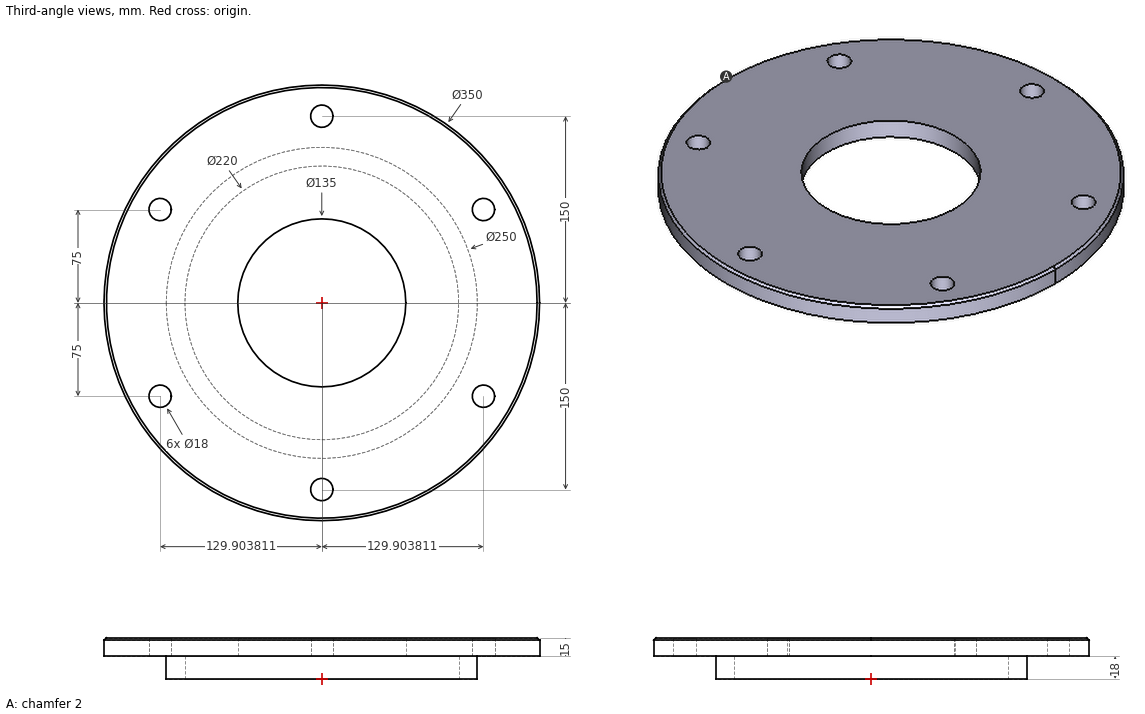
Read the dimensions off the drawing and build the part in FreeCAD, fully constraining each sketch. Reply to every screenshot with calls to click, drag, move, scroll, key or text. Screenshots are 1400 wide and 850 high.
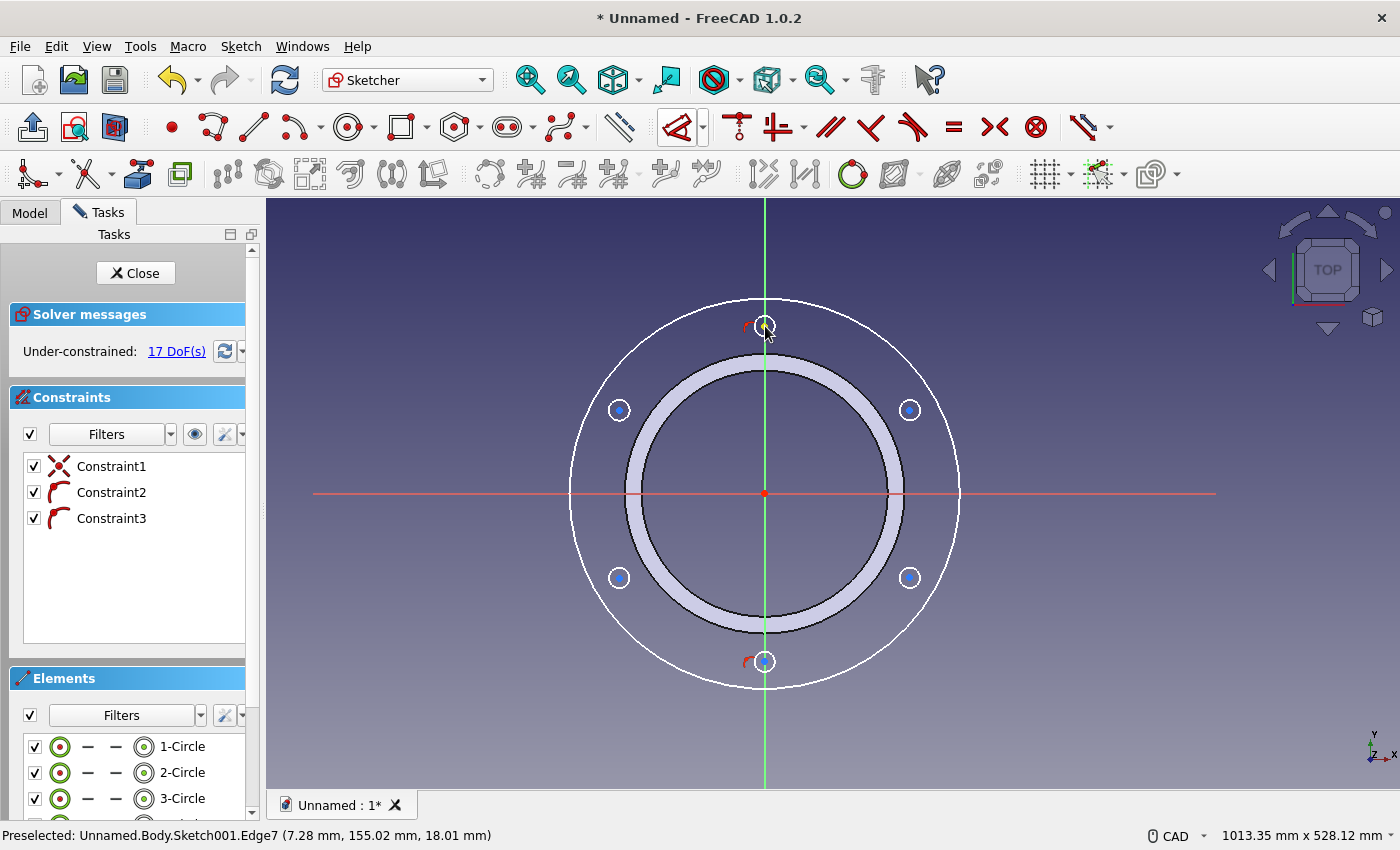
scroll(626, 571, up, 2)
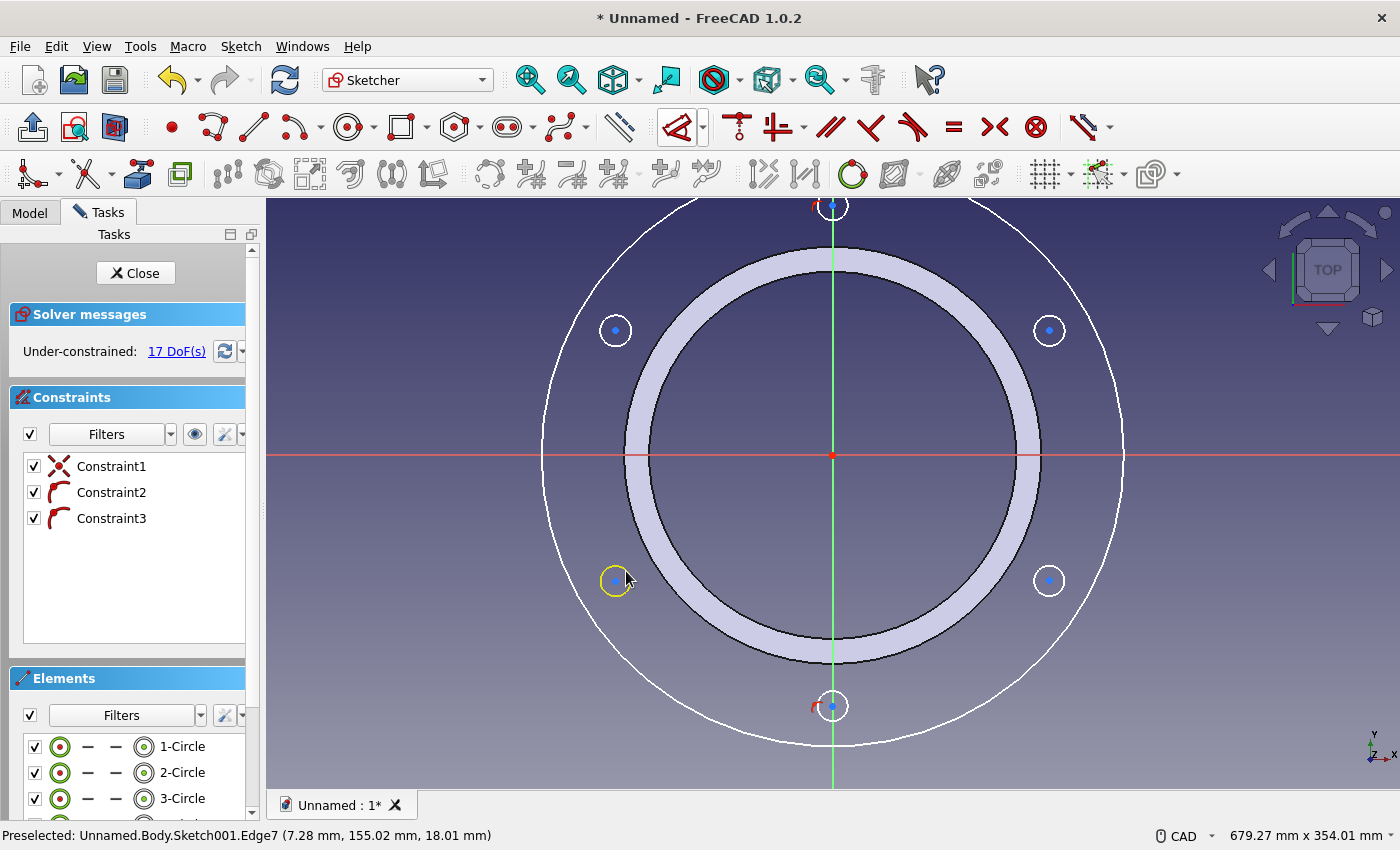
click(626, 570)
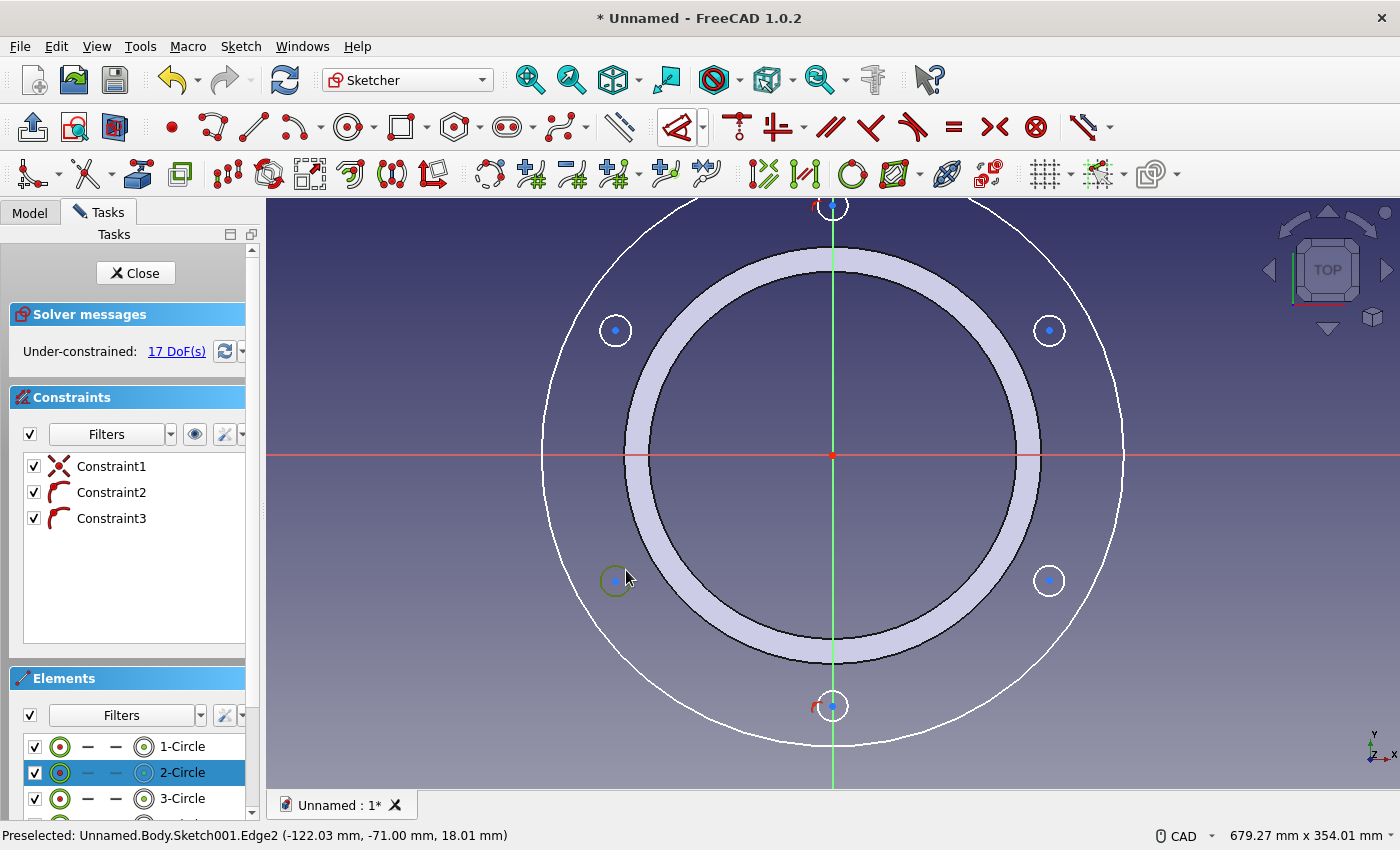
scroll(843, 695, up, 2)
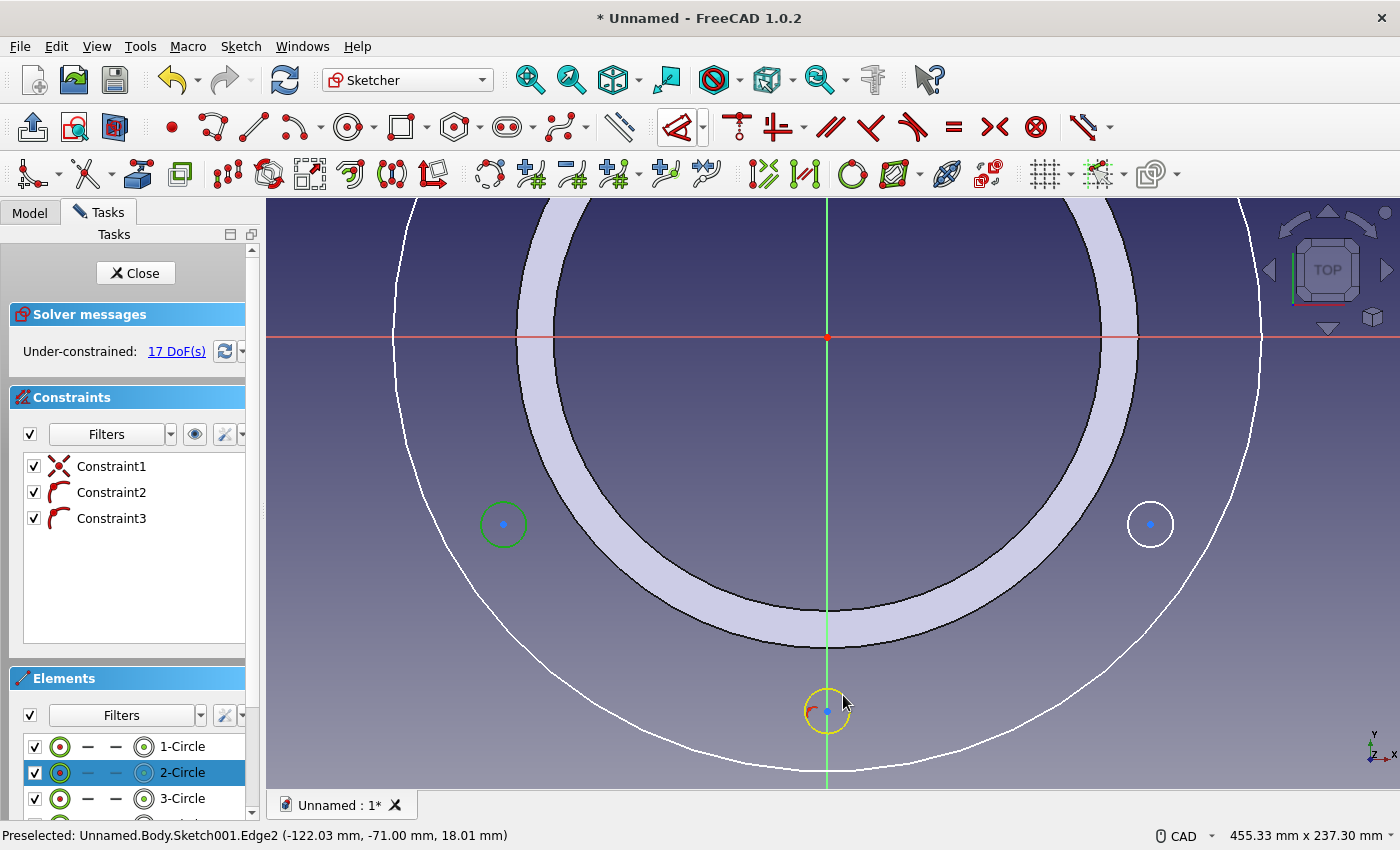
click(843, 695)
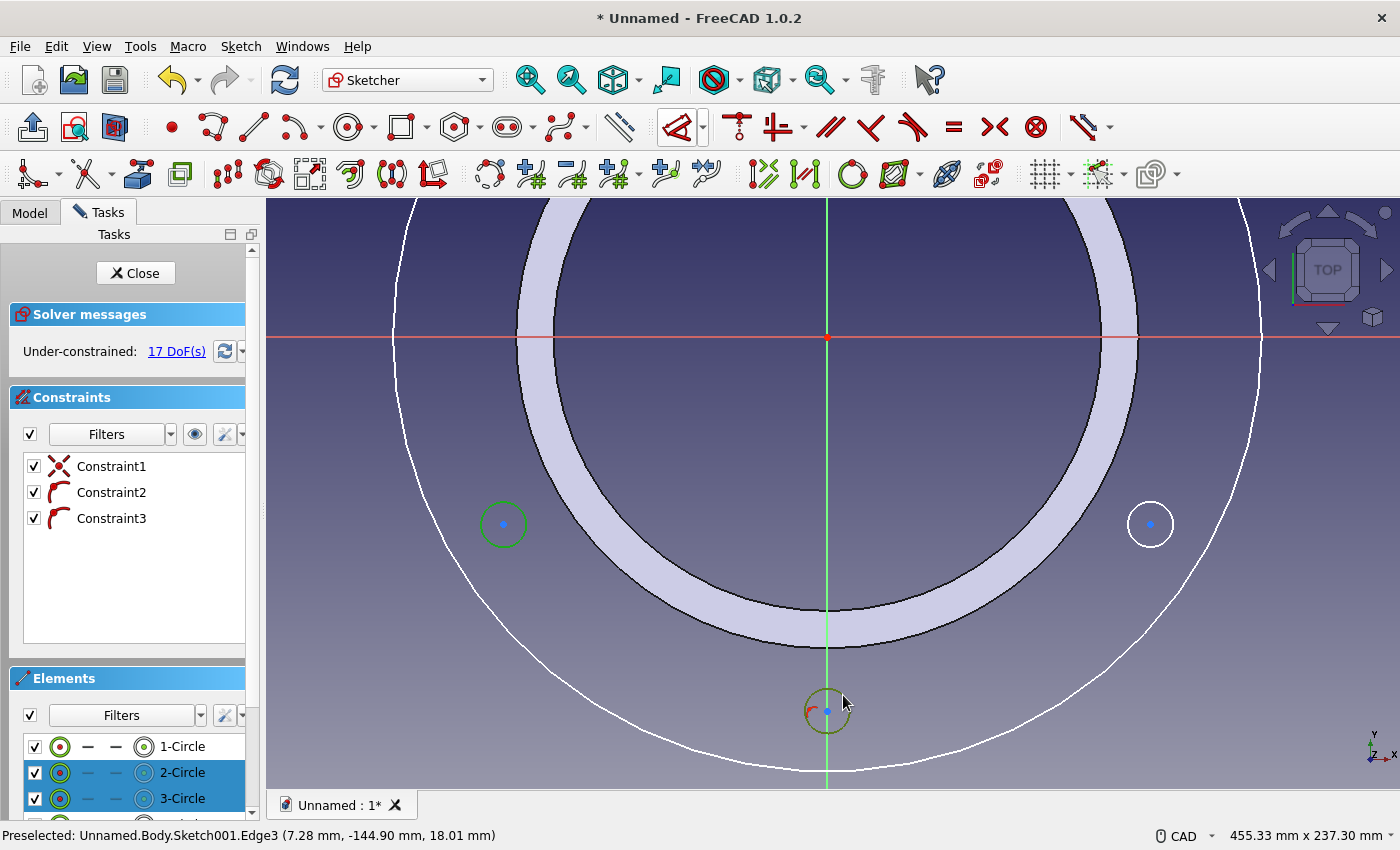
click(1166, 508)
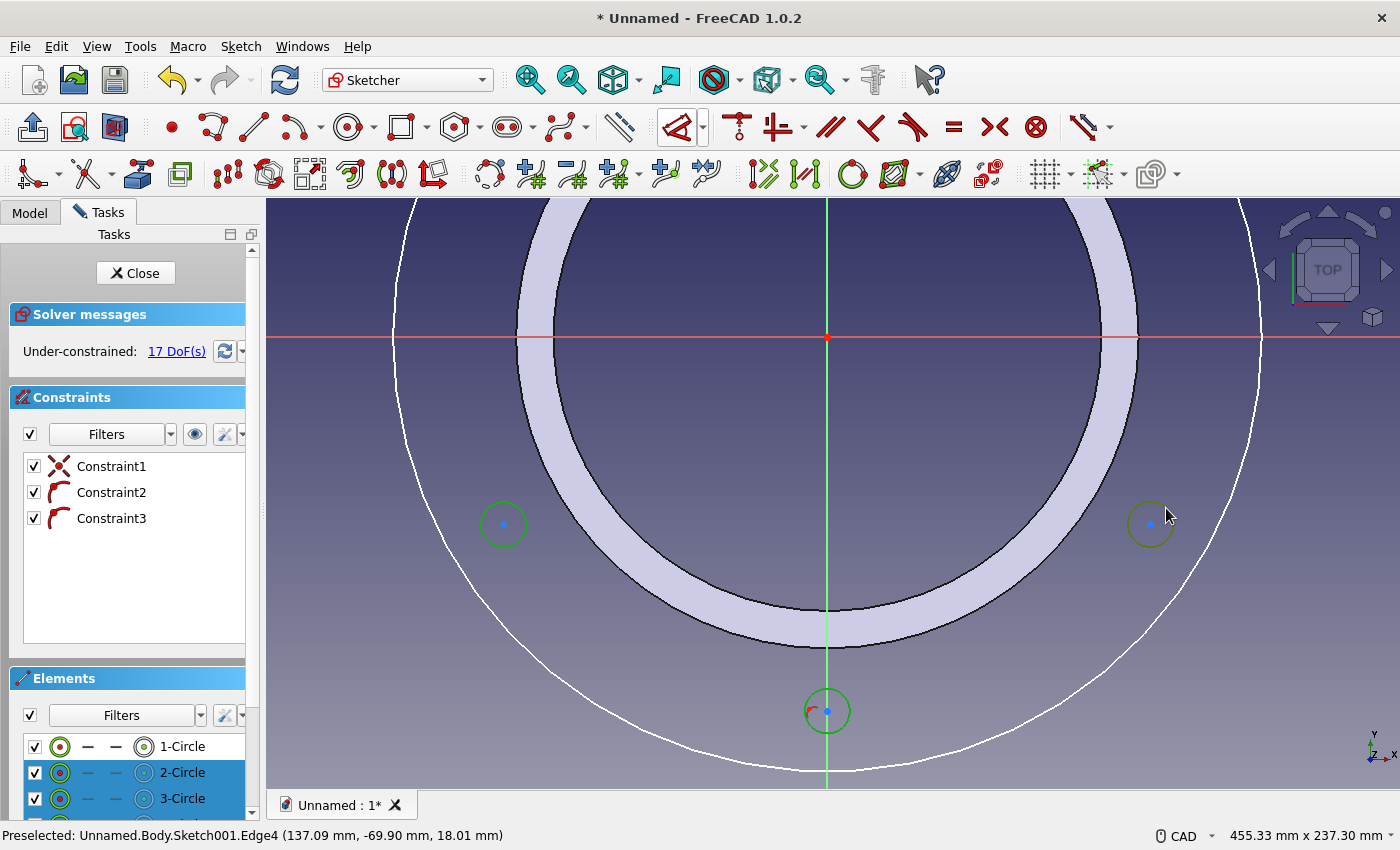
scroll(713, 621, down, 4)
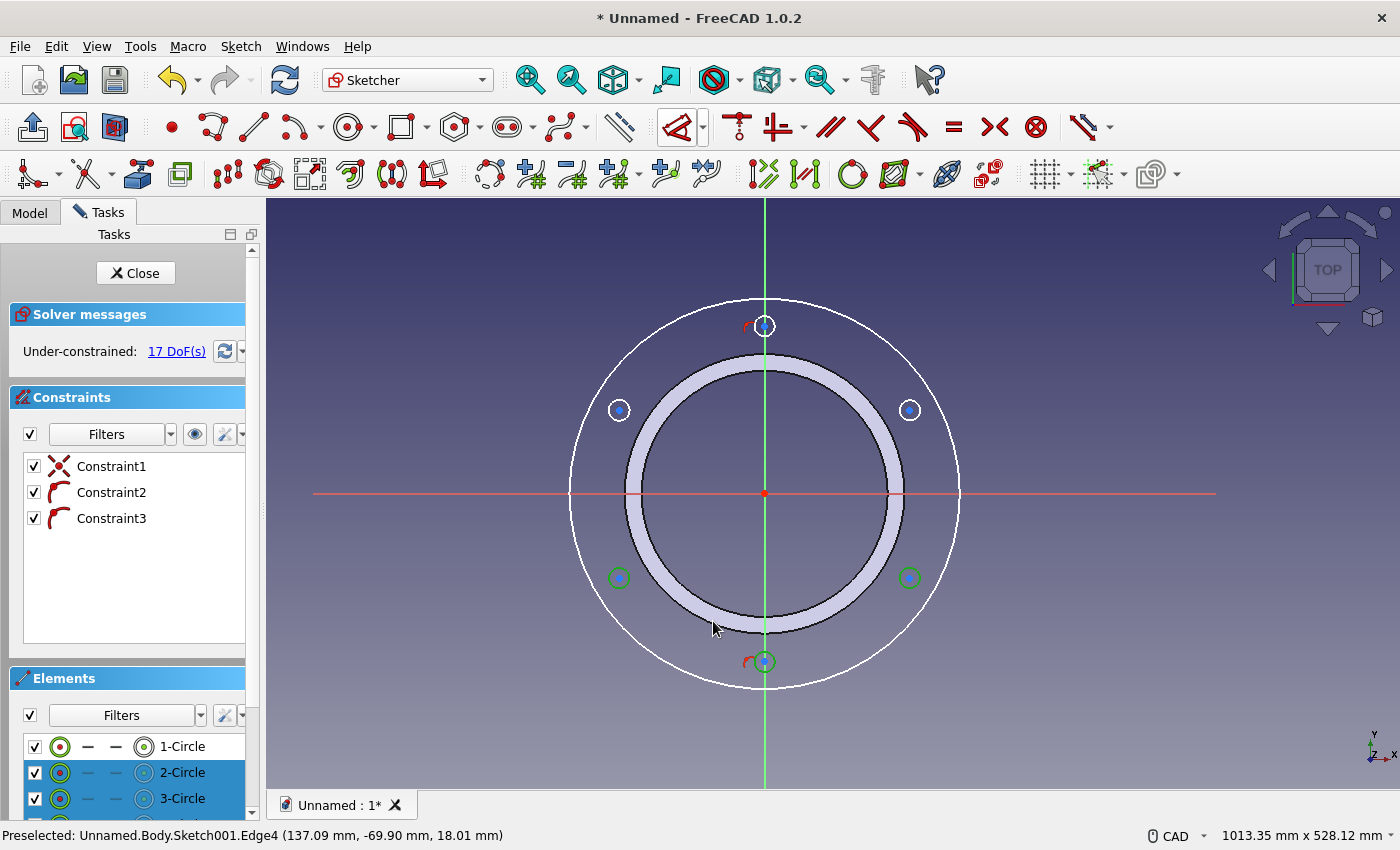
scroll(626, 403, up, 2)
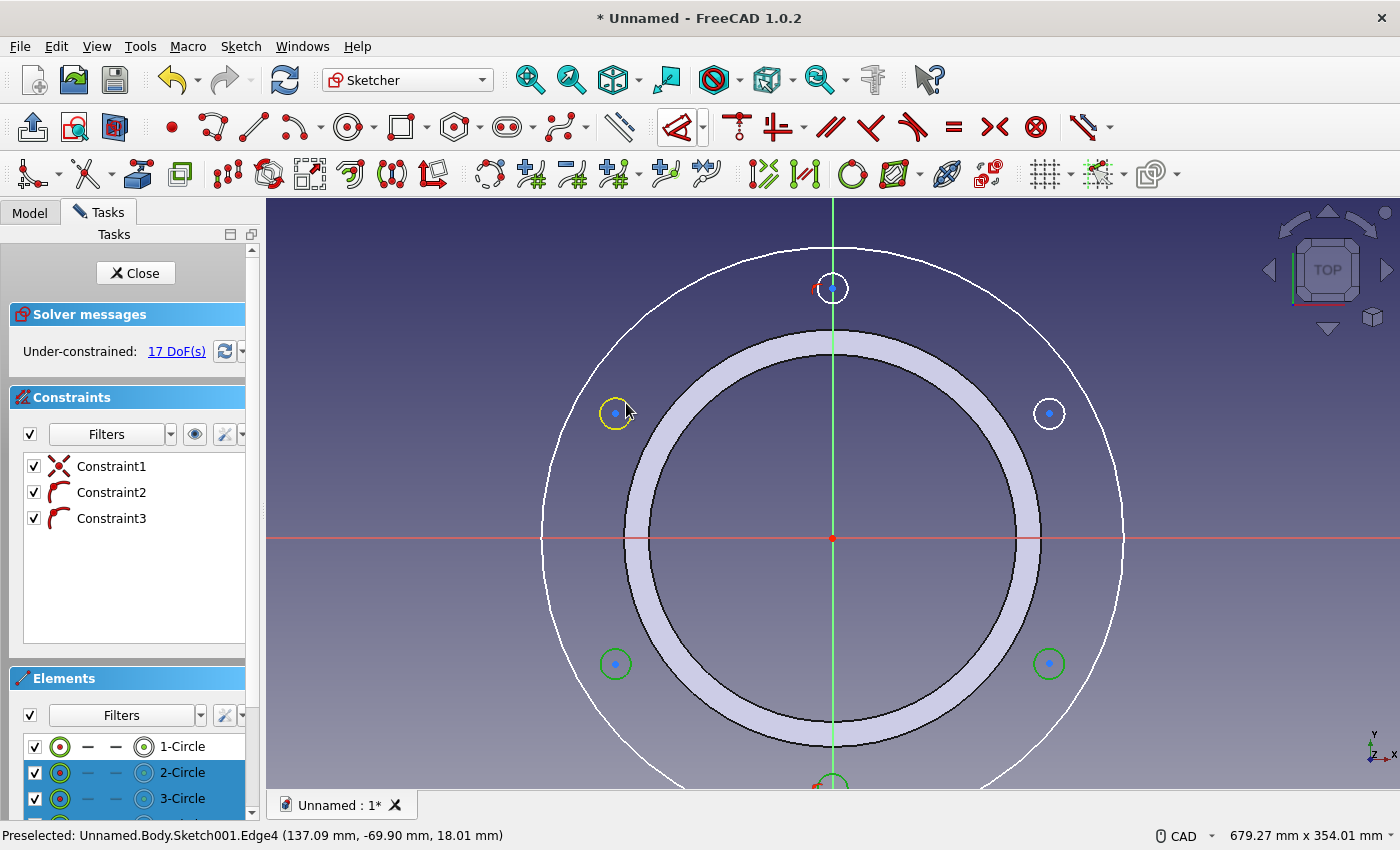
click(627, 403)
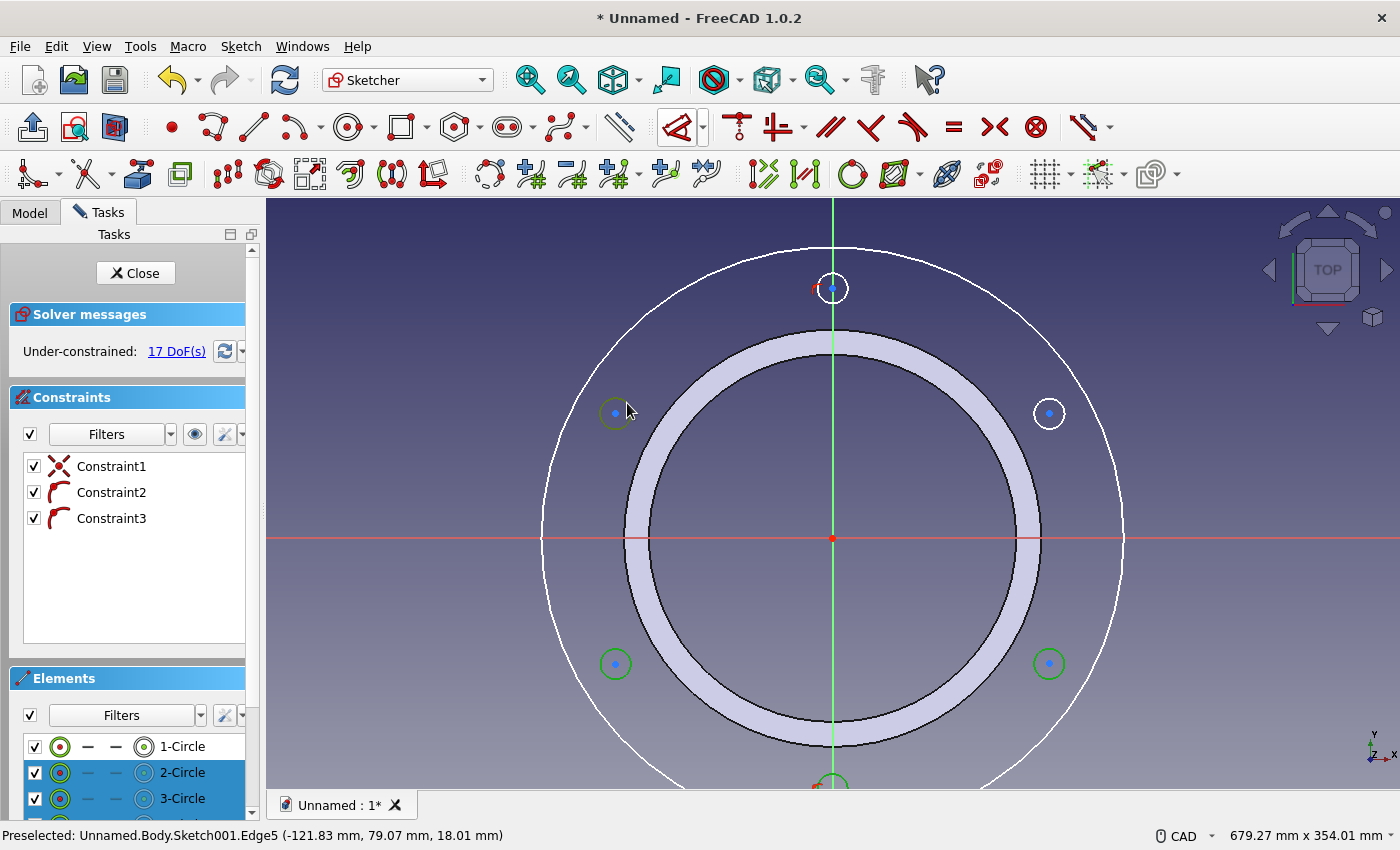
click(1060, 403)